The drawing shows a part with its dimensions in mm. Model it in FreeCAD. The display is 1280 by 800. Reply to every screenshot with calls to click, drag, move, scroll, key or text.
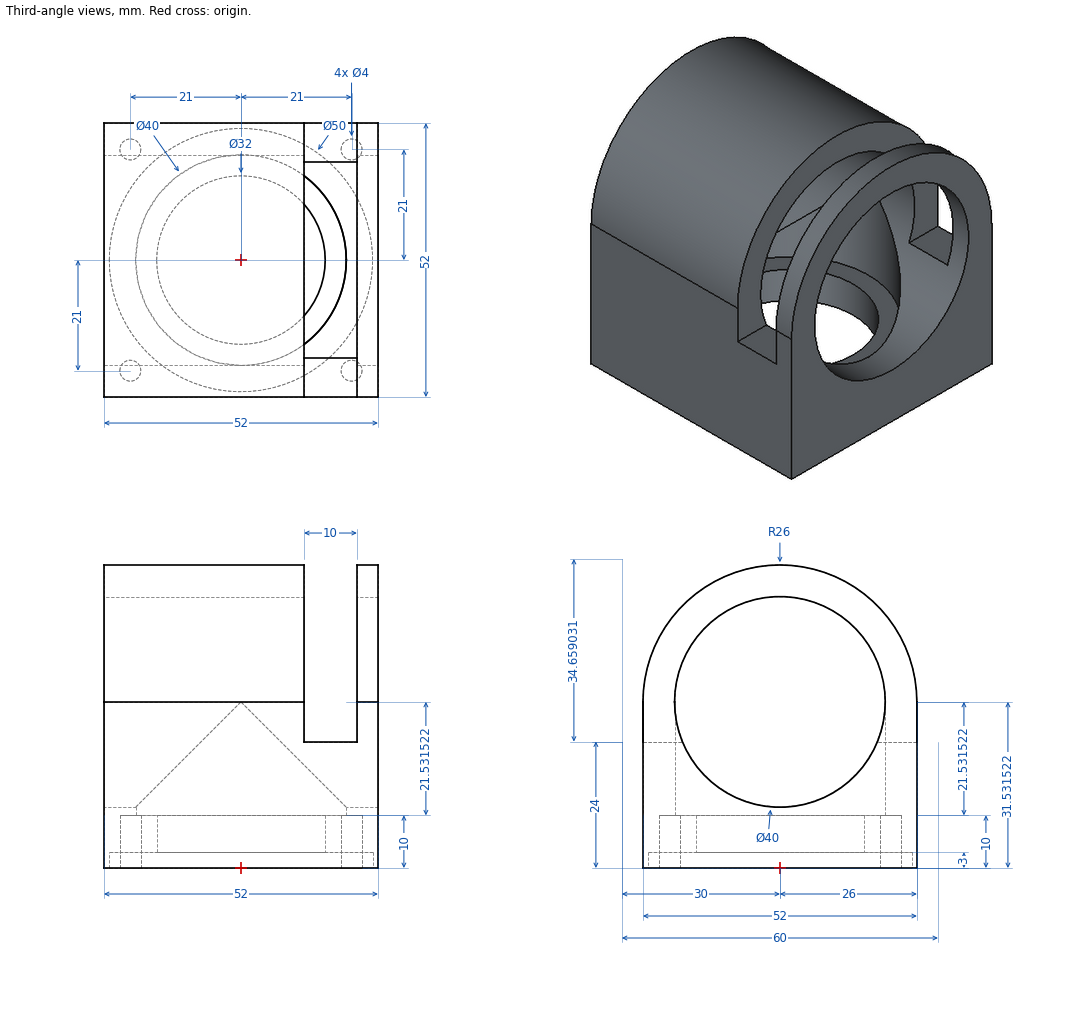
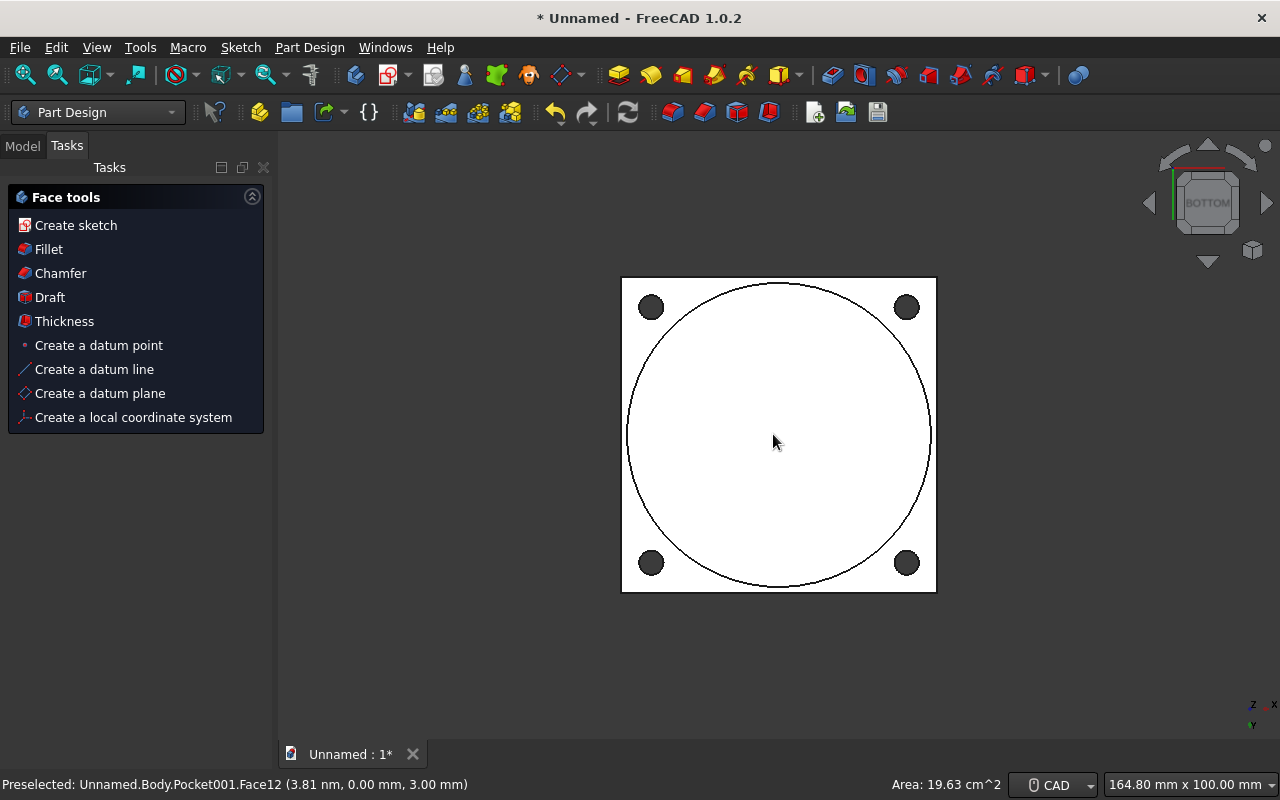
click(388, 76)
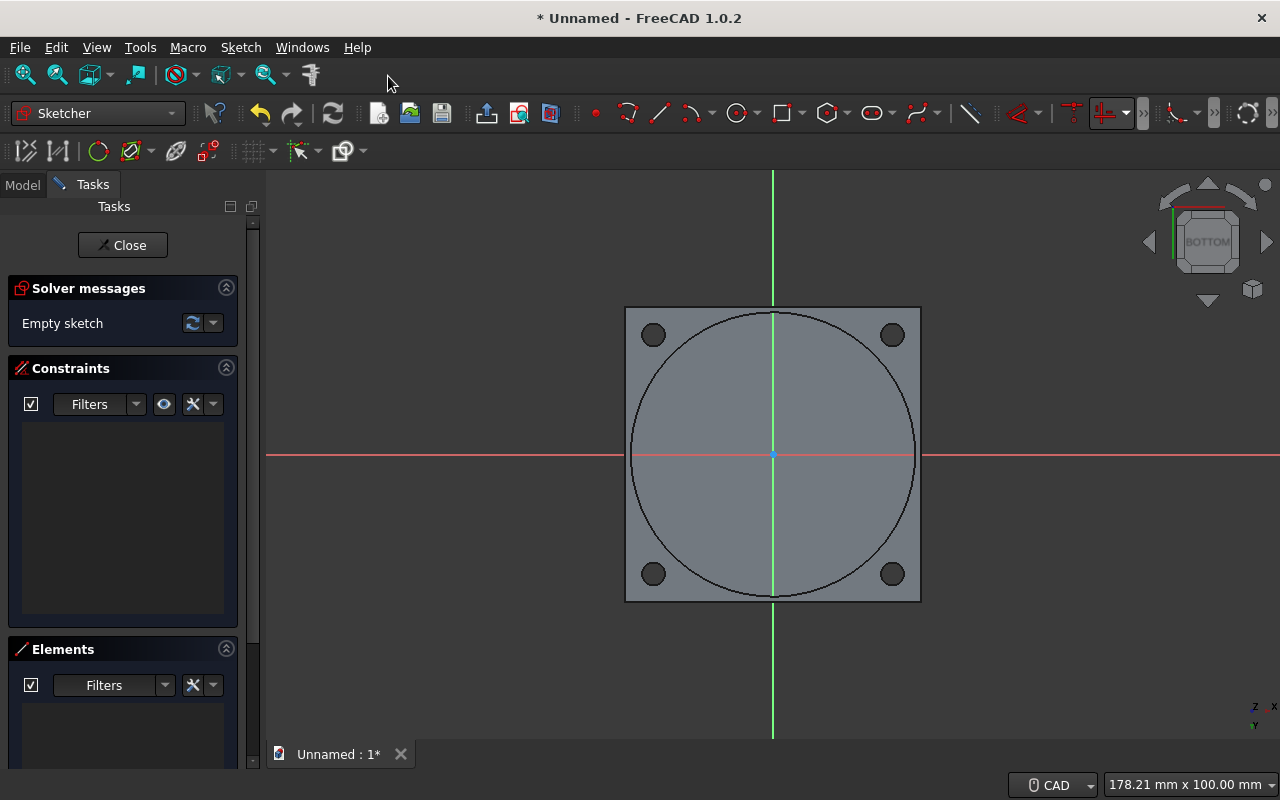
click(552, 114)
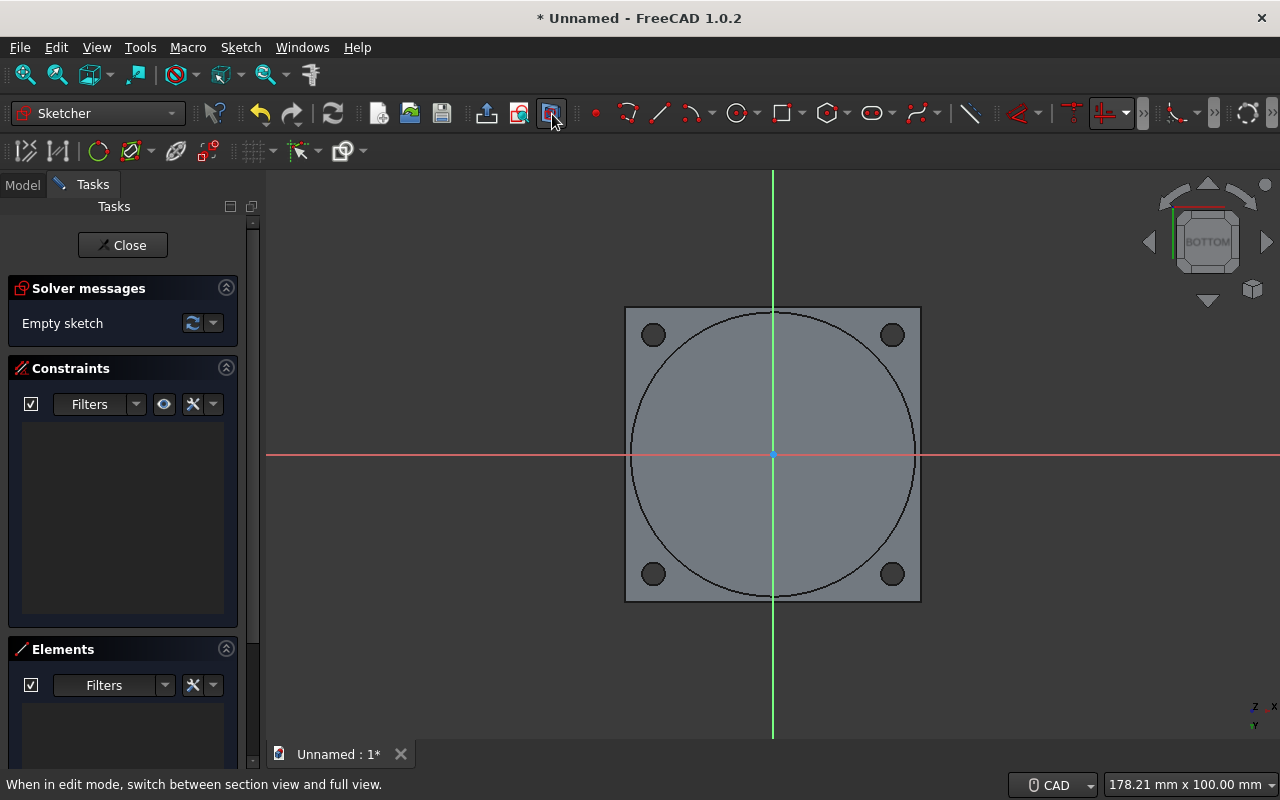
scroll(856, 454, up, 3)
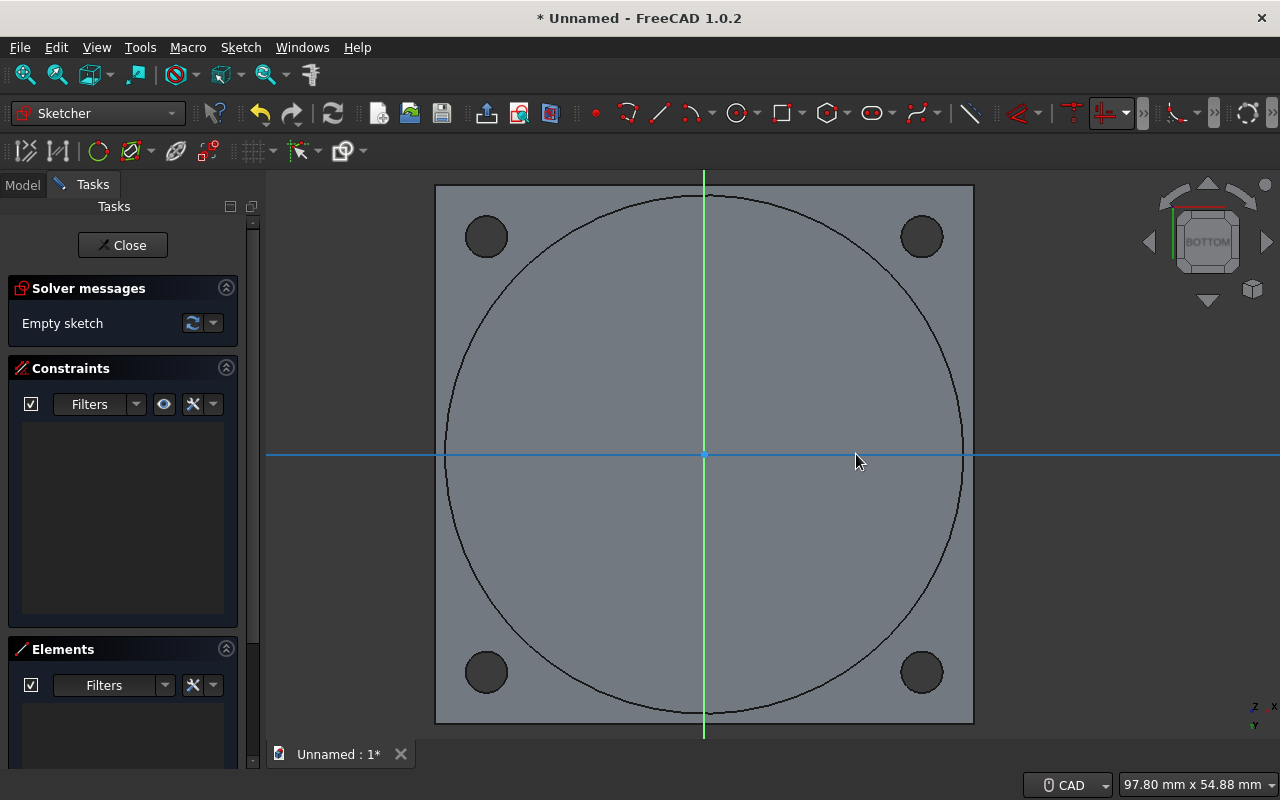
click(738, 114)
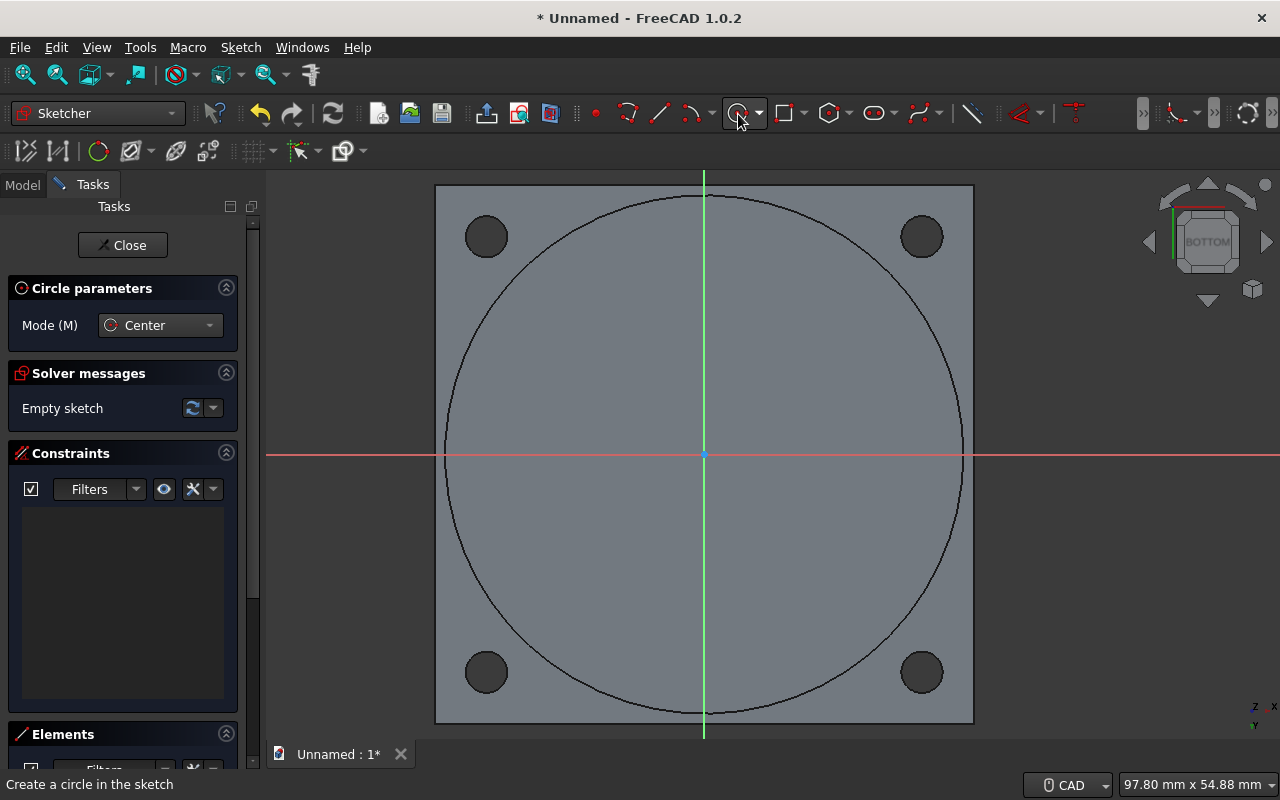
click(704, 454)
click(822, 337)
key(Escape)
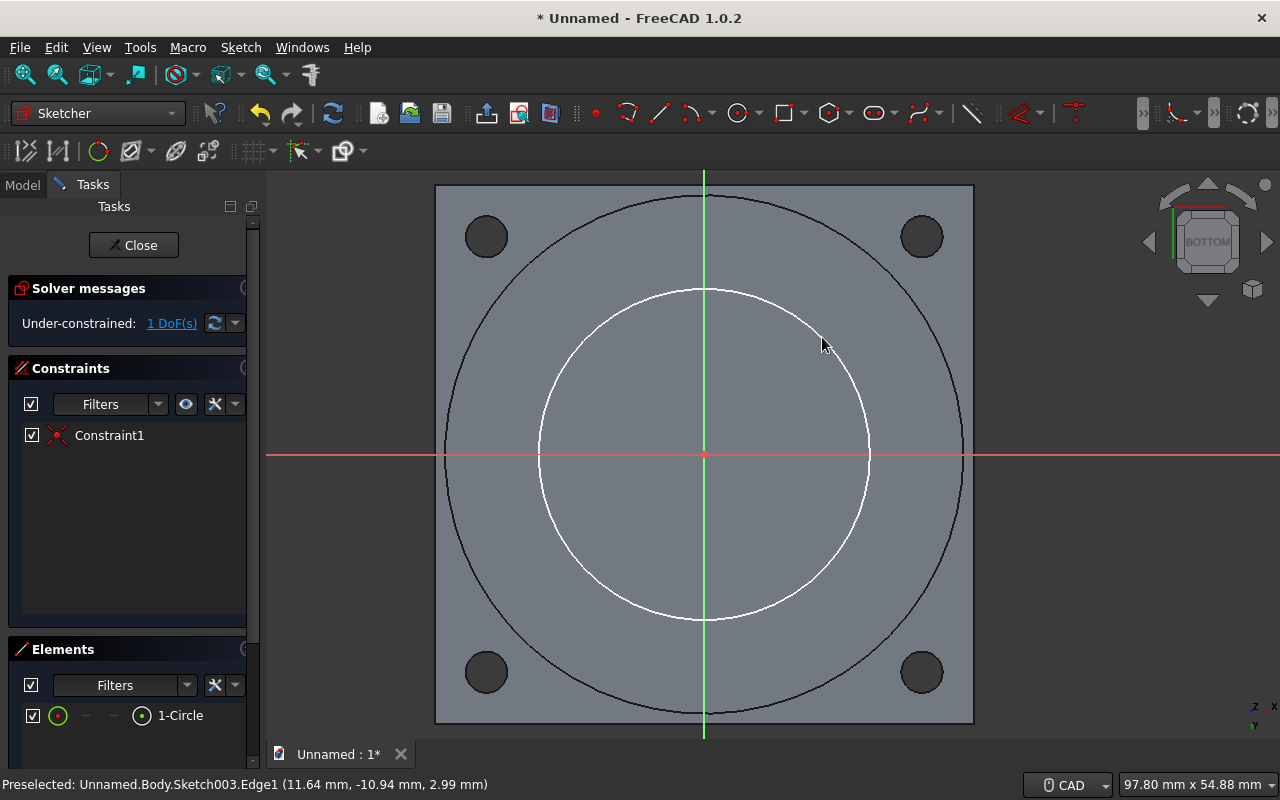
click(1020, 114)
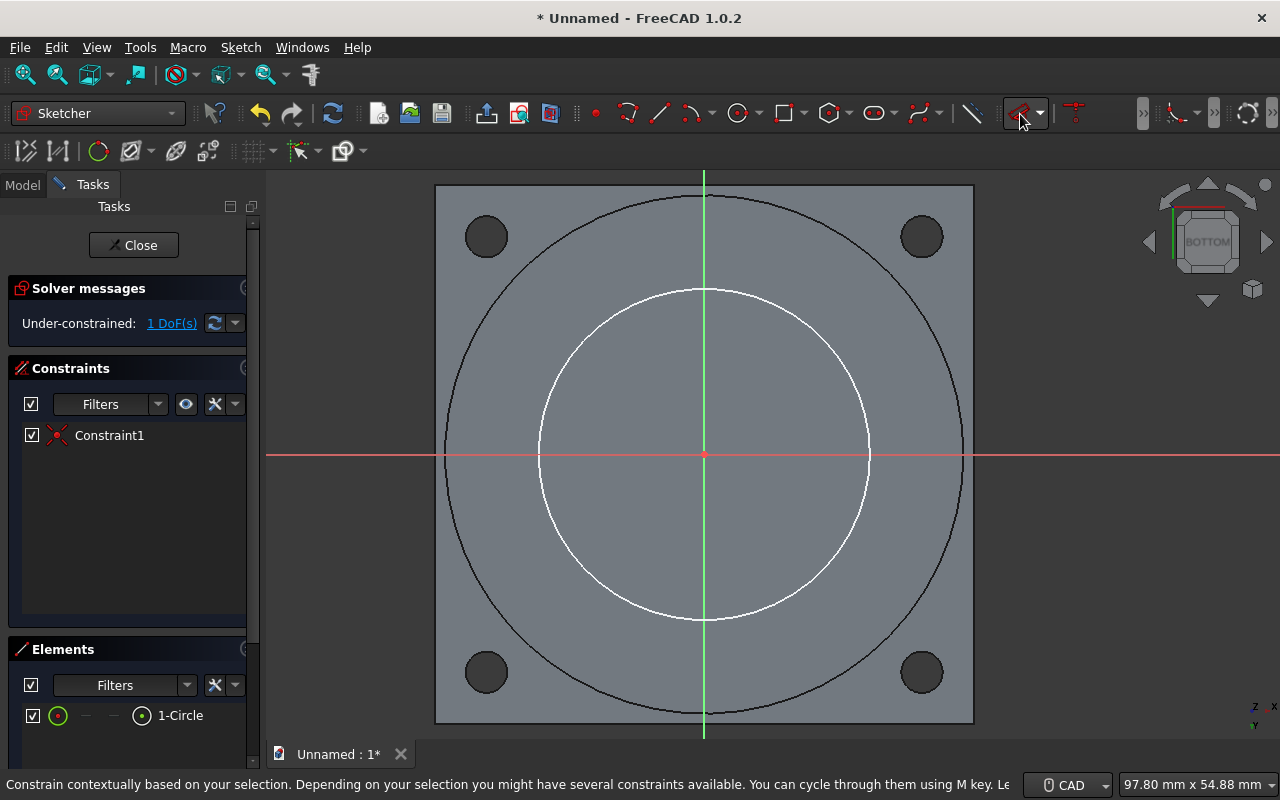
click(821, 337)
click(844, 314)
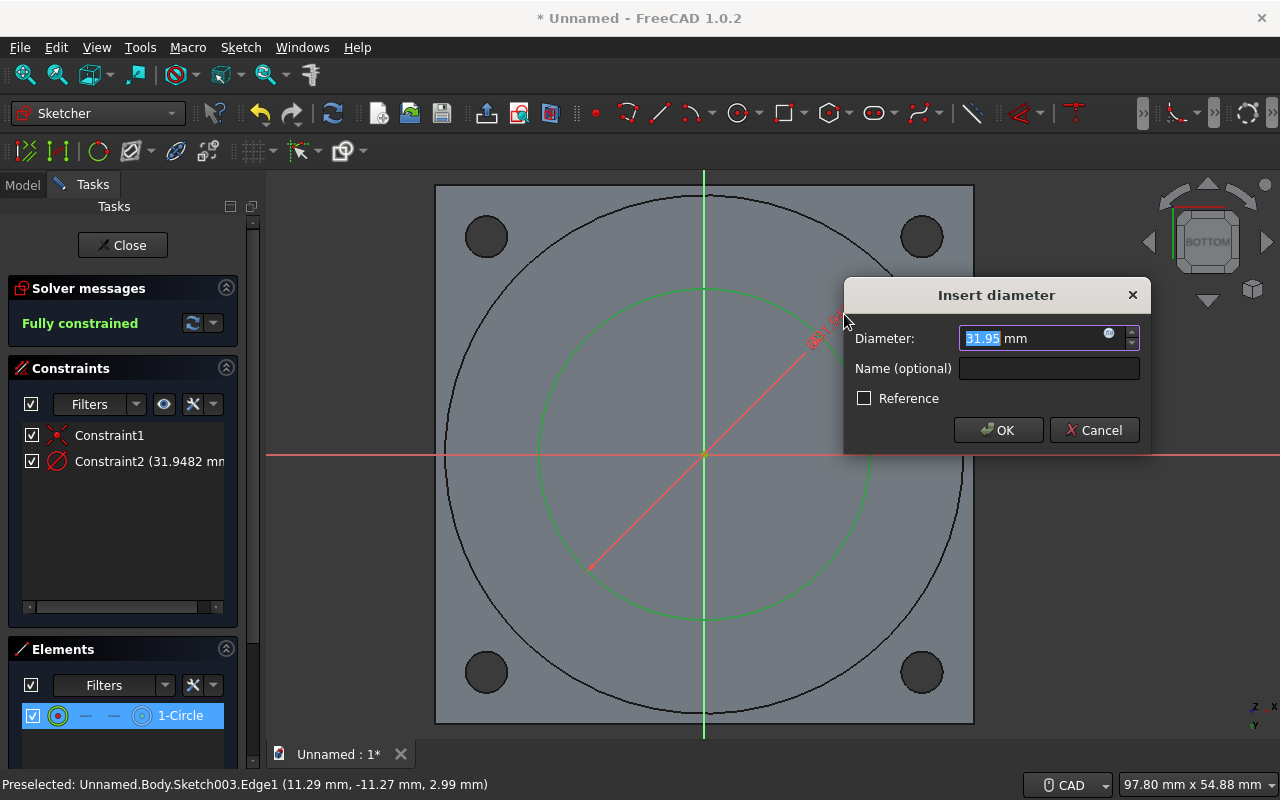
text(32)
key(Return)
key(Escape)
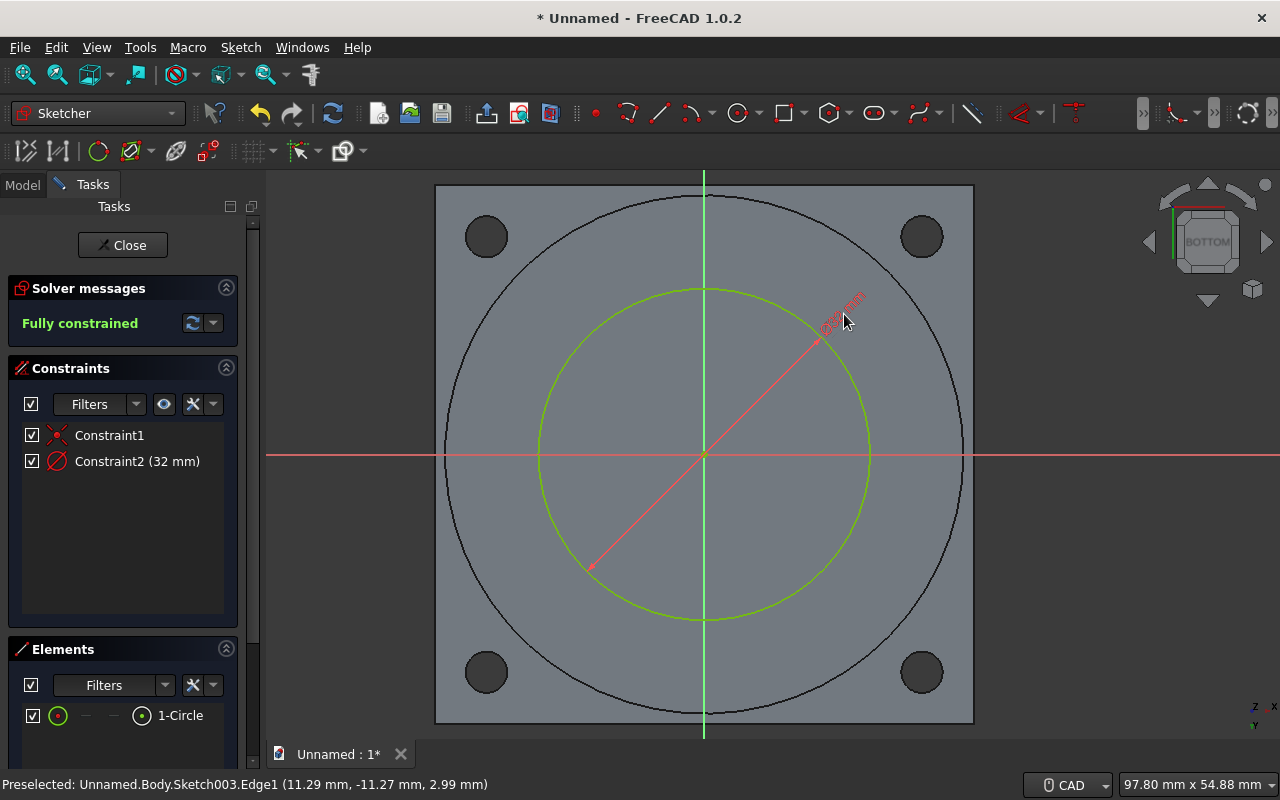
click(123, 245)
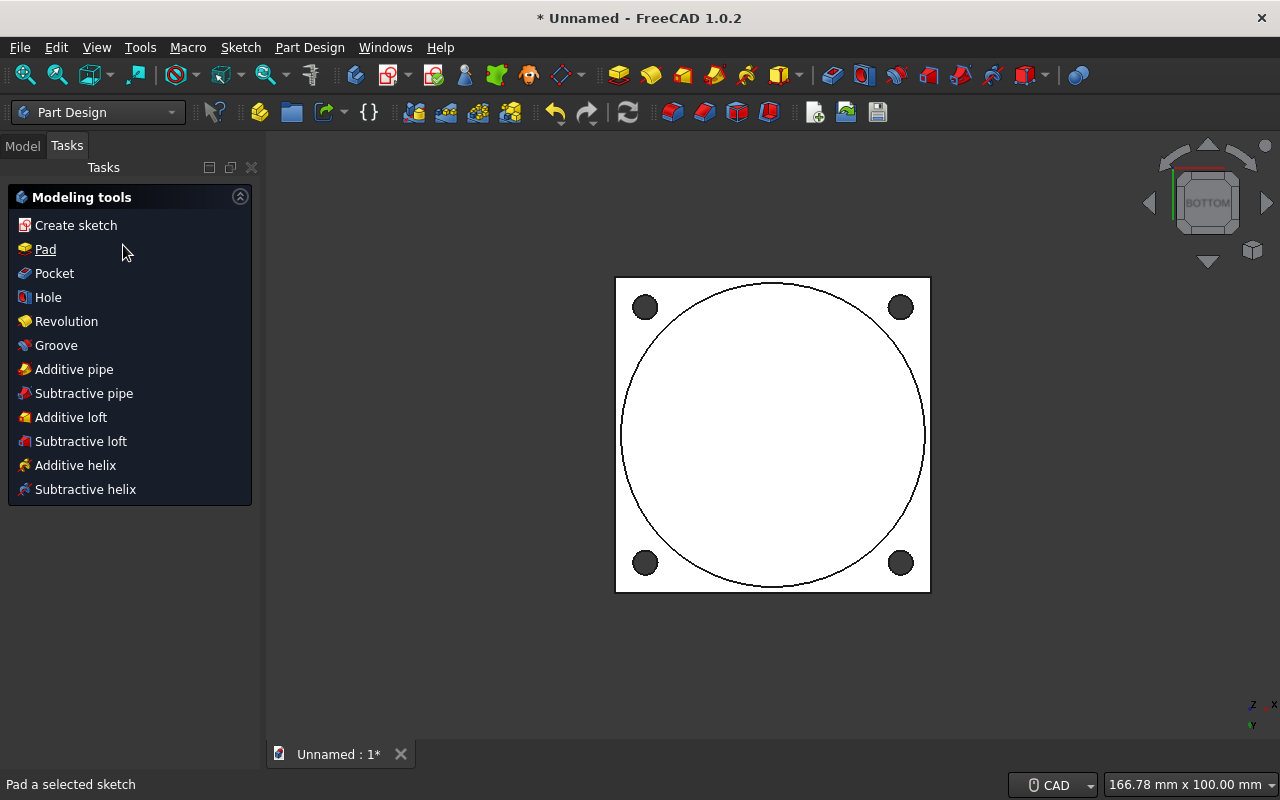
click(834, 76)